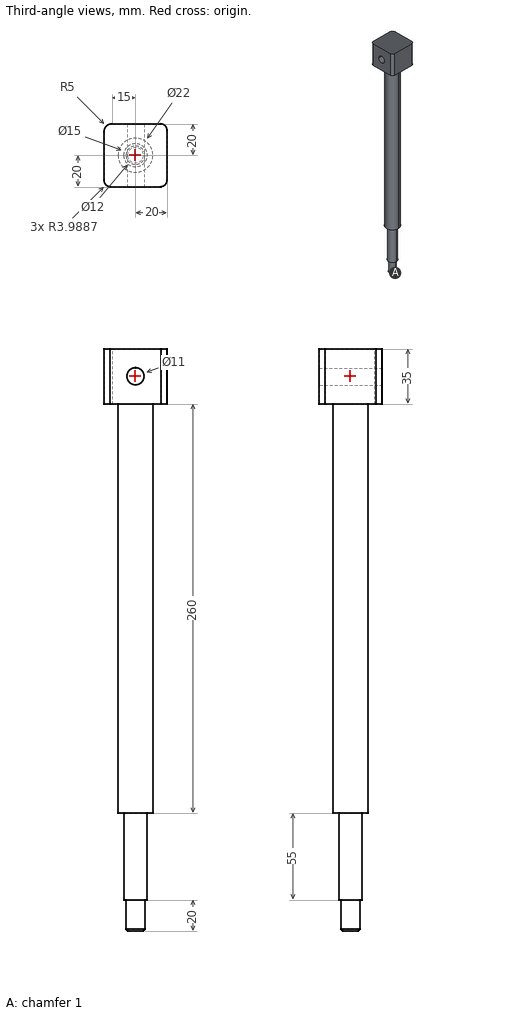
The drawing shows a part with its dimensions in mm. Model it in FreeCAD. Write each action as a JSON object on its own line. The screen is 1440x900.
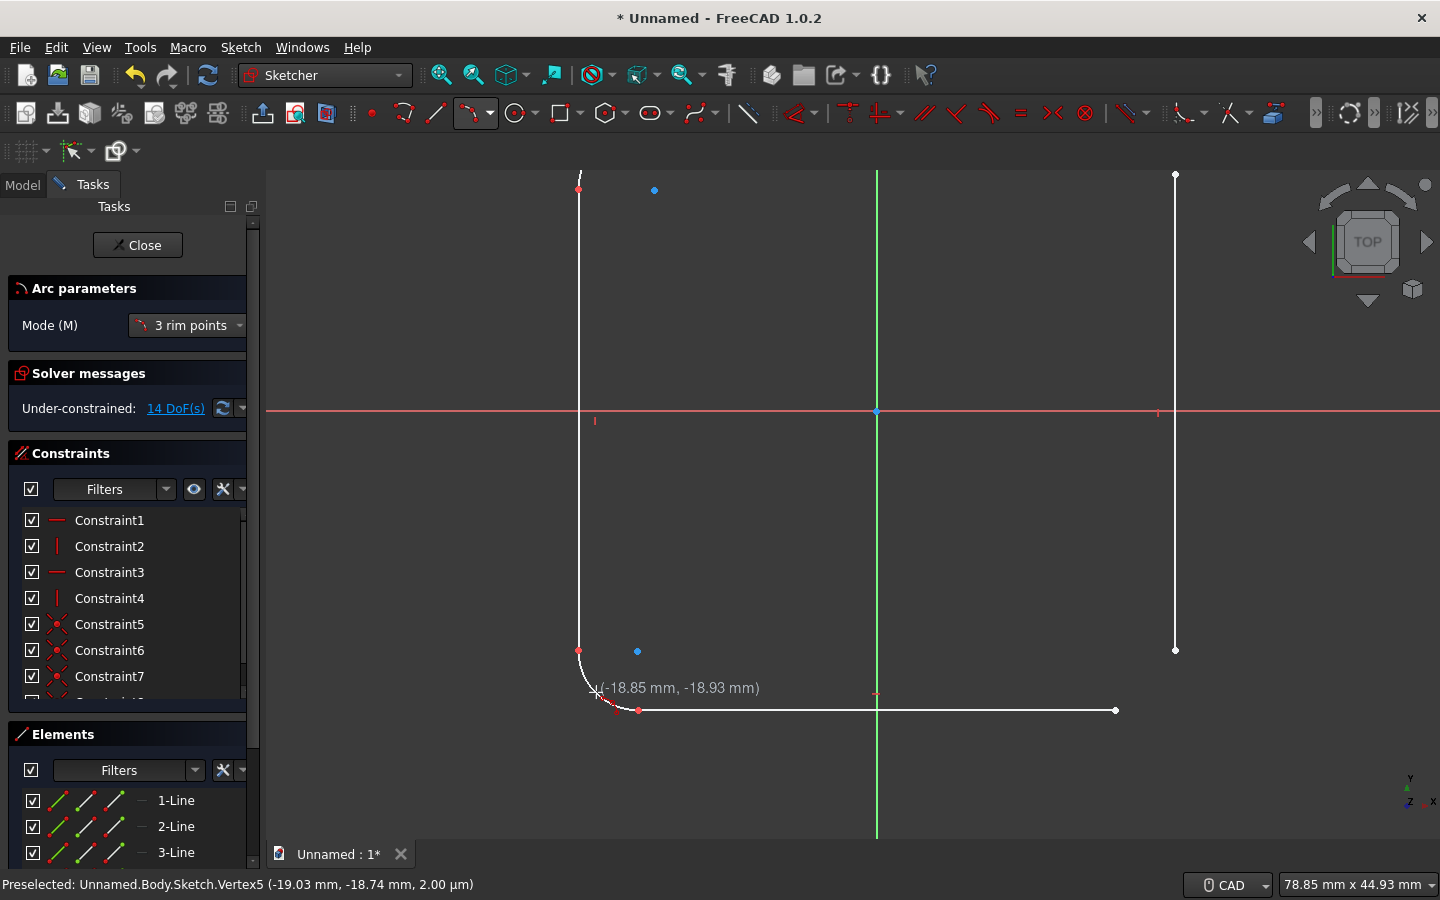
{"action": "left_click", "coordinate": [1116, 710]}
{"action": "left_click", "coordinate": [1175, 651]}
{"action": "left_click", "coordinate": [1157, 692]}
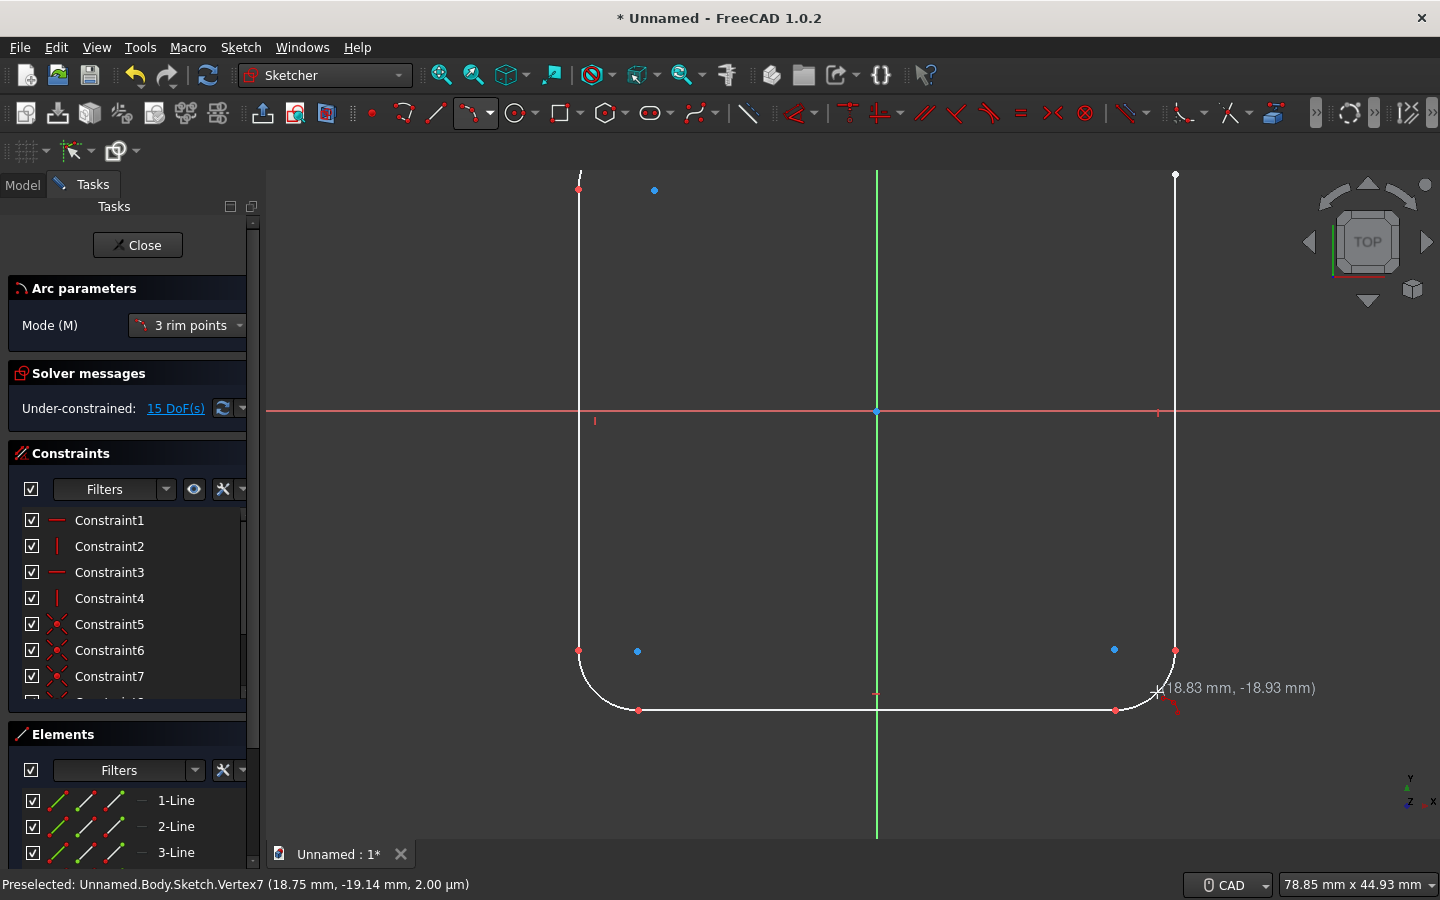
{"action": "scroll", "coordinate": [597, 694], "scroll_direction": "down", "scroll_amount": 2}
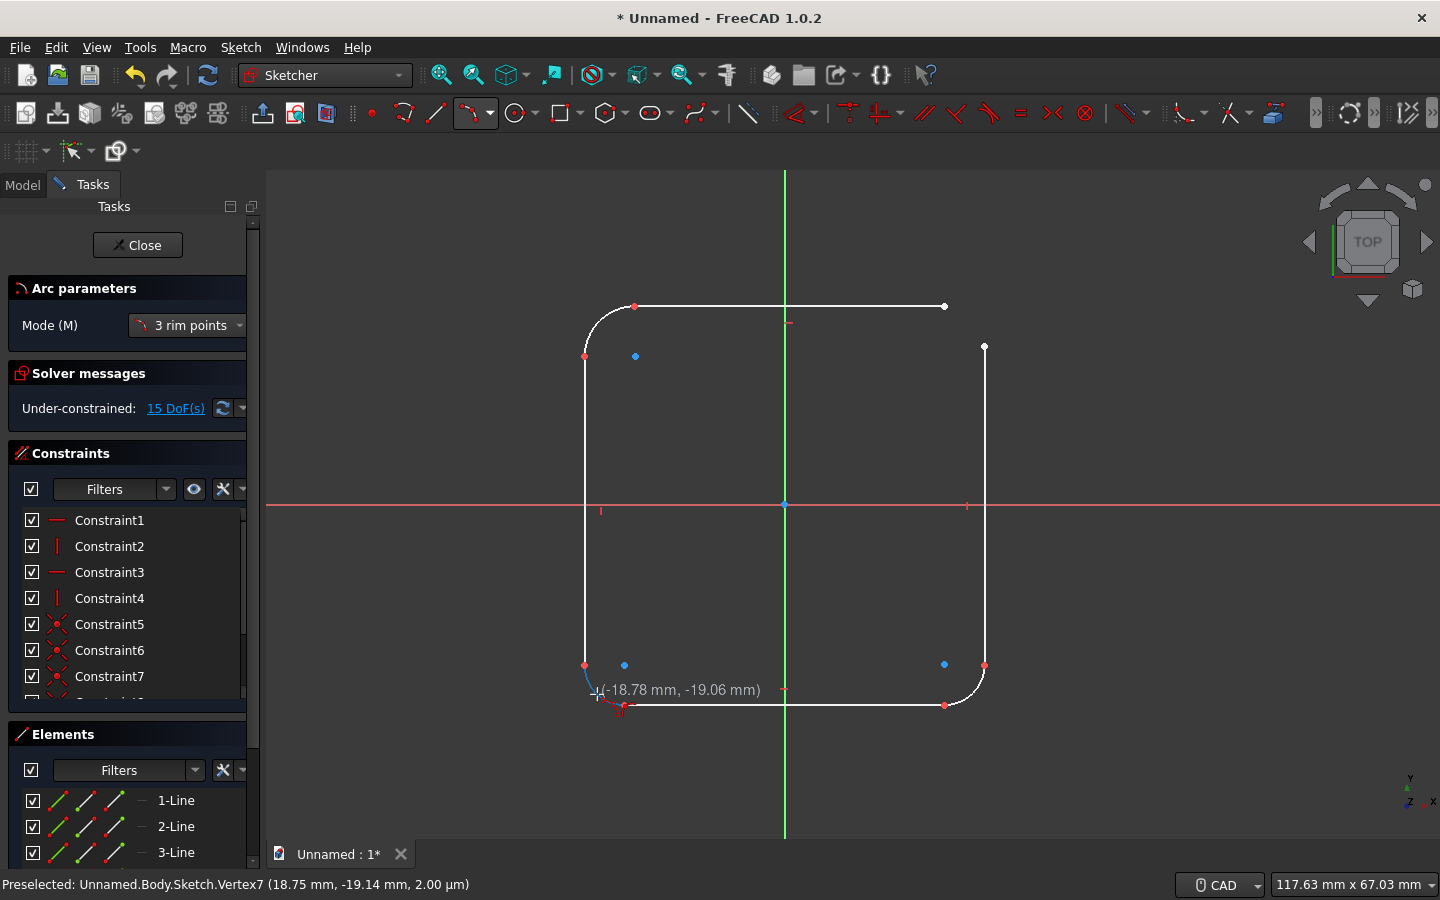
{"action": "left_click", "coordinate": [985, 346]}
{"action": "left_click", "coordinate": [945, 306]}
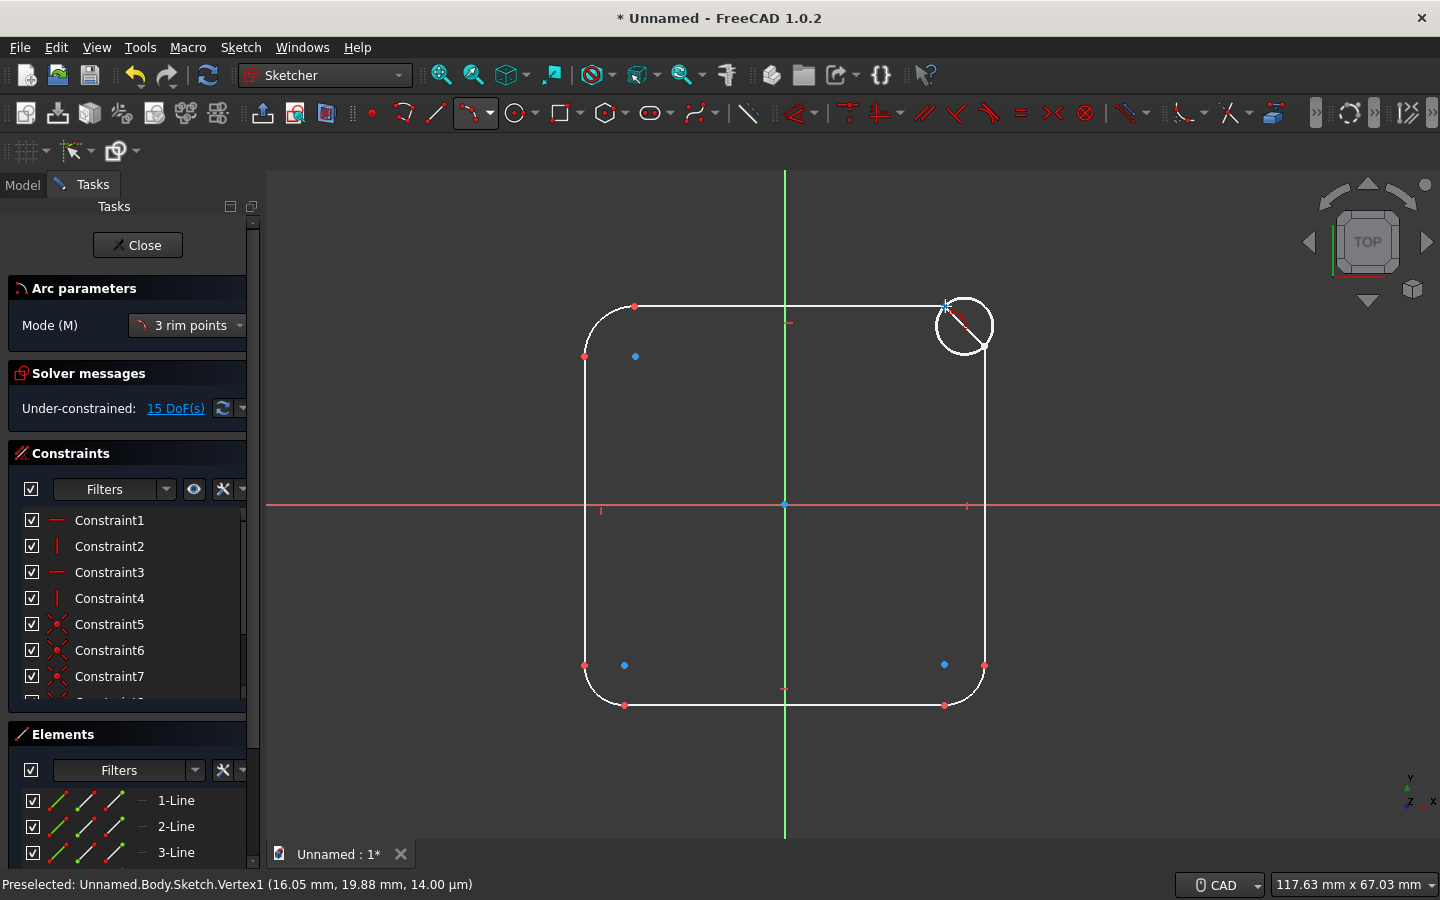
{"action": "scroll", "coordinate": [972, 317], "scroll_direction": "up", "scroll_amount": 2}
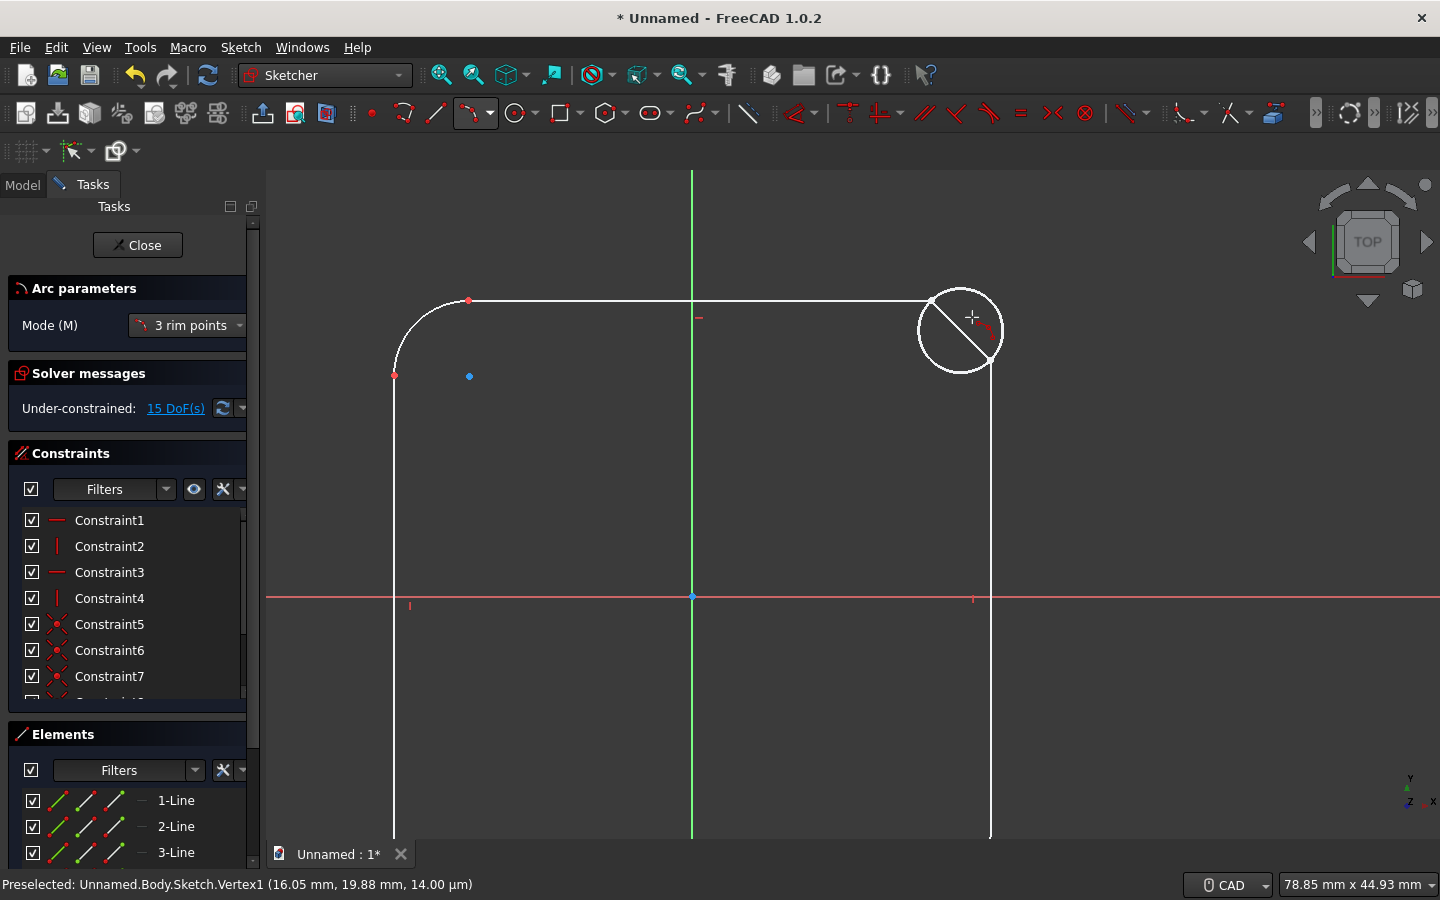
{"action": "left_click", "coordinate": [972, 316]}
{"action": "key", "text": "Escape"}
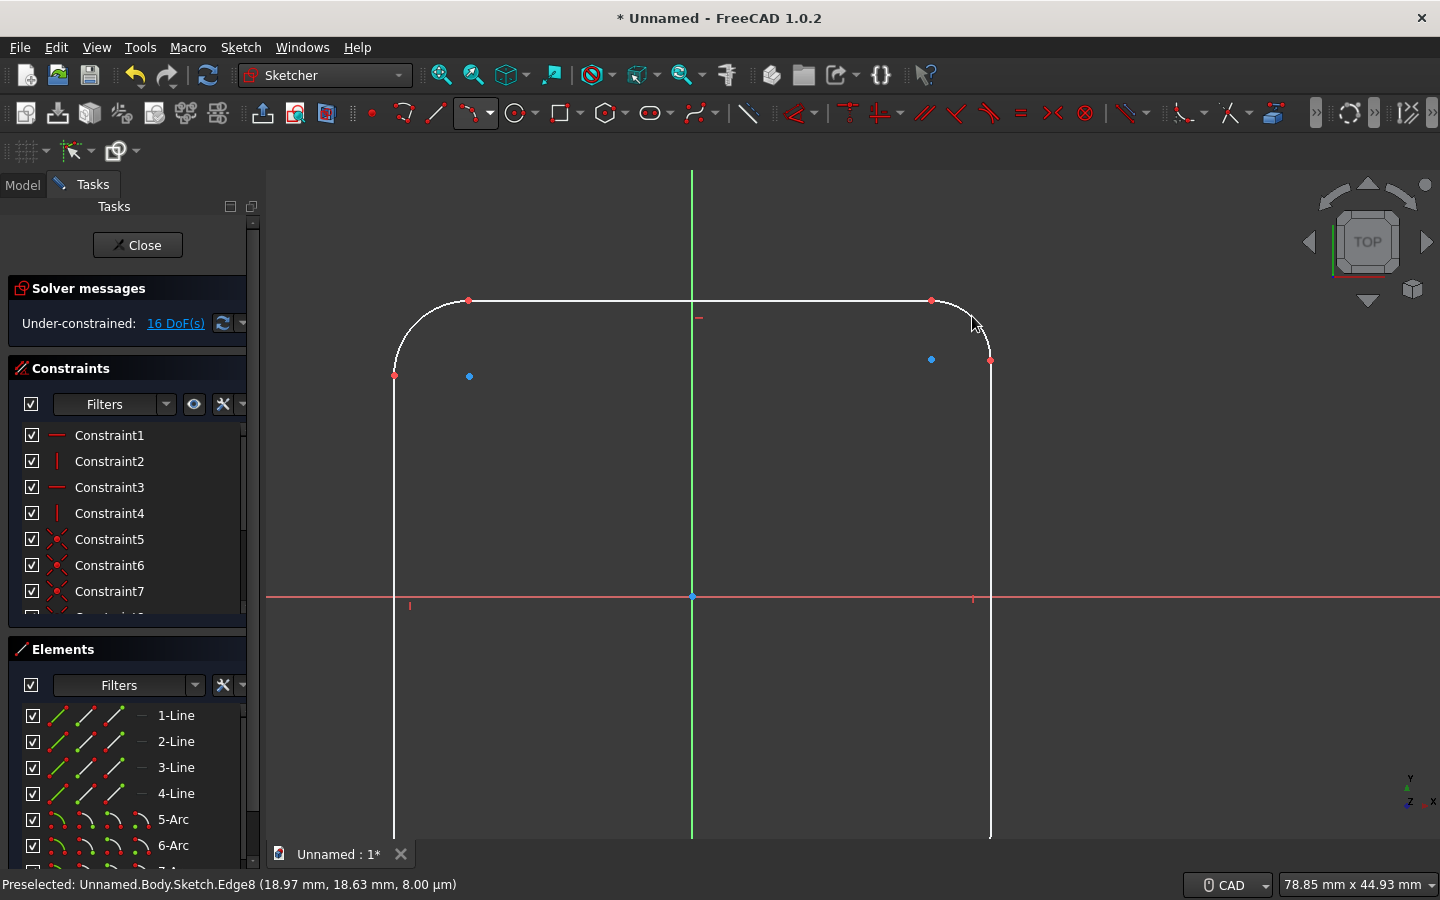
{"action": "left_click", "coordinate": [792, 301]}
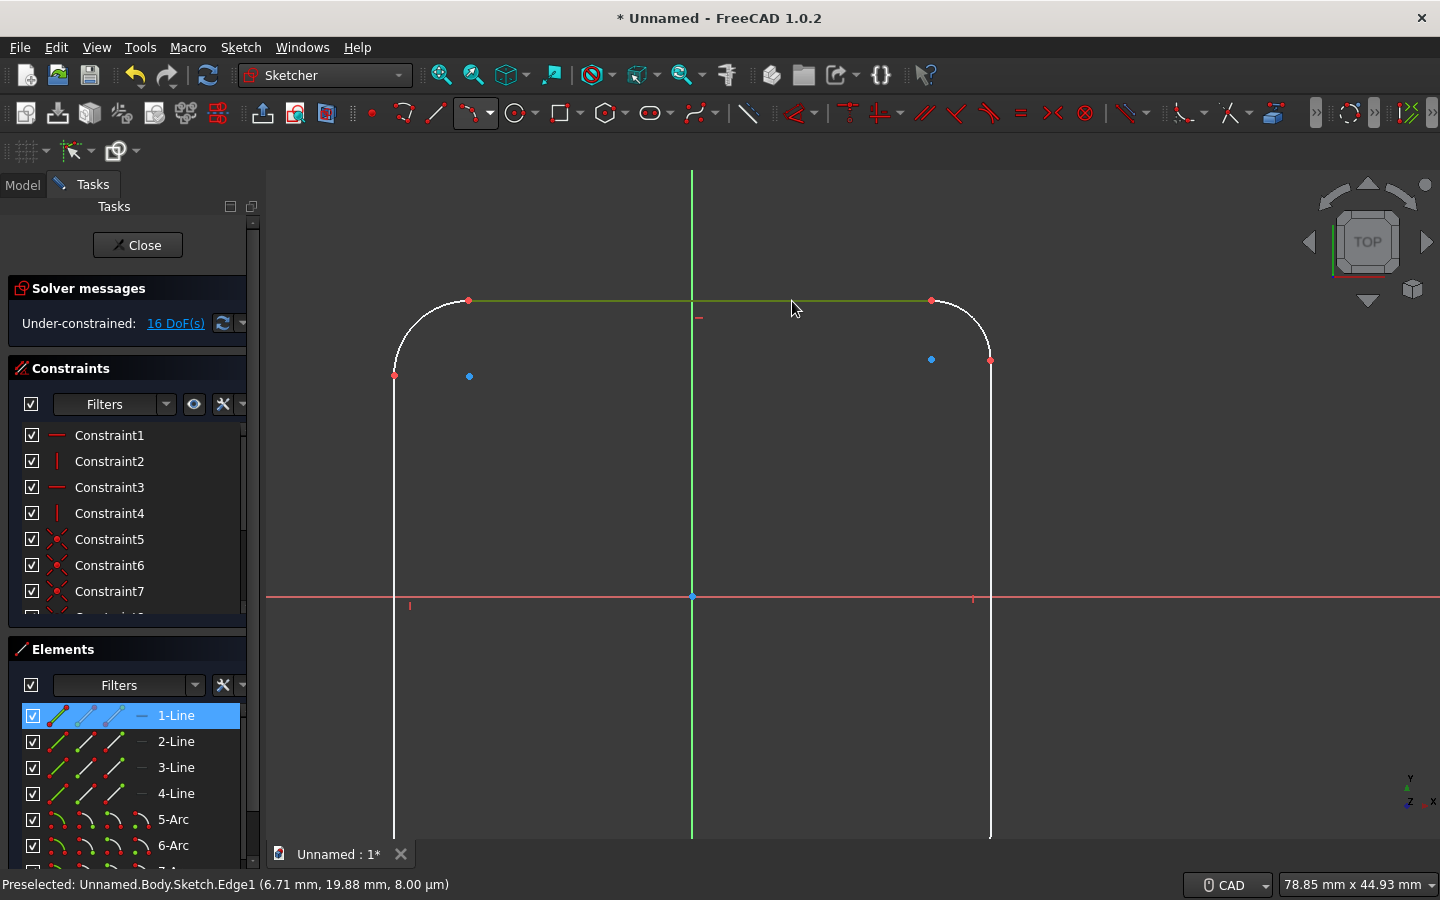
{"action": "left_click", "coordinate": [435, 309]}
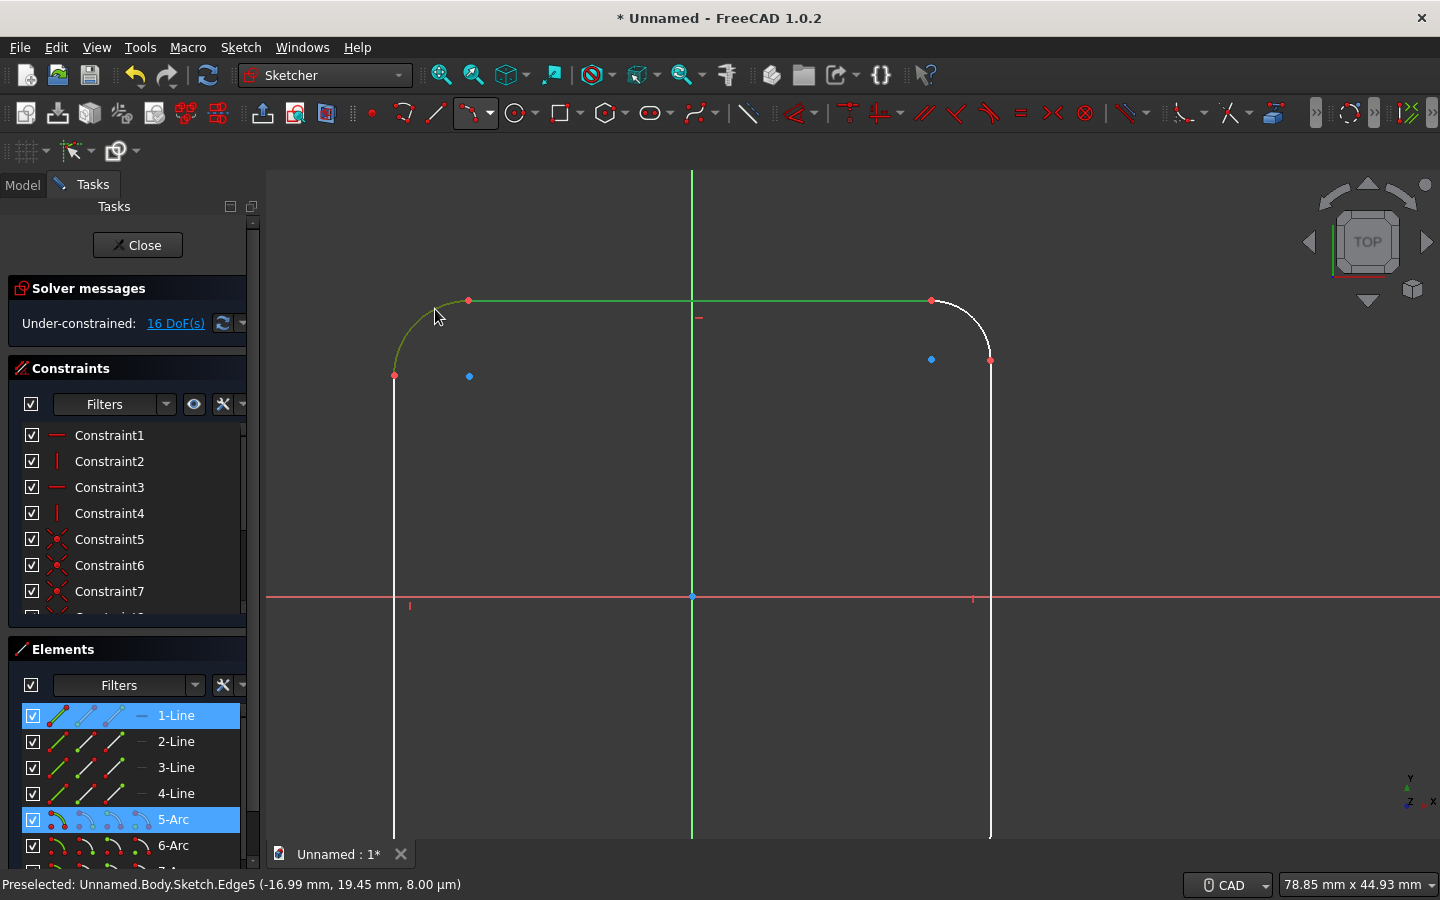
{"action": "key", "text": "t"}